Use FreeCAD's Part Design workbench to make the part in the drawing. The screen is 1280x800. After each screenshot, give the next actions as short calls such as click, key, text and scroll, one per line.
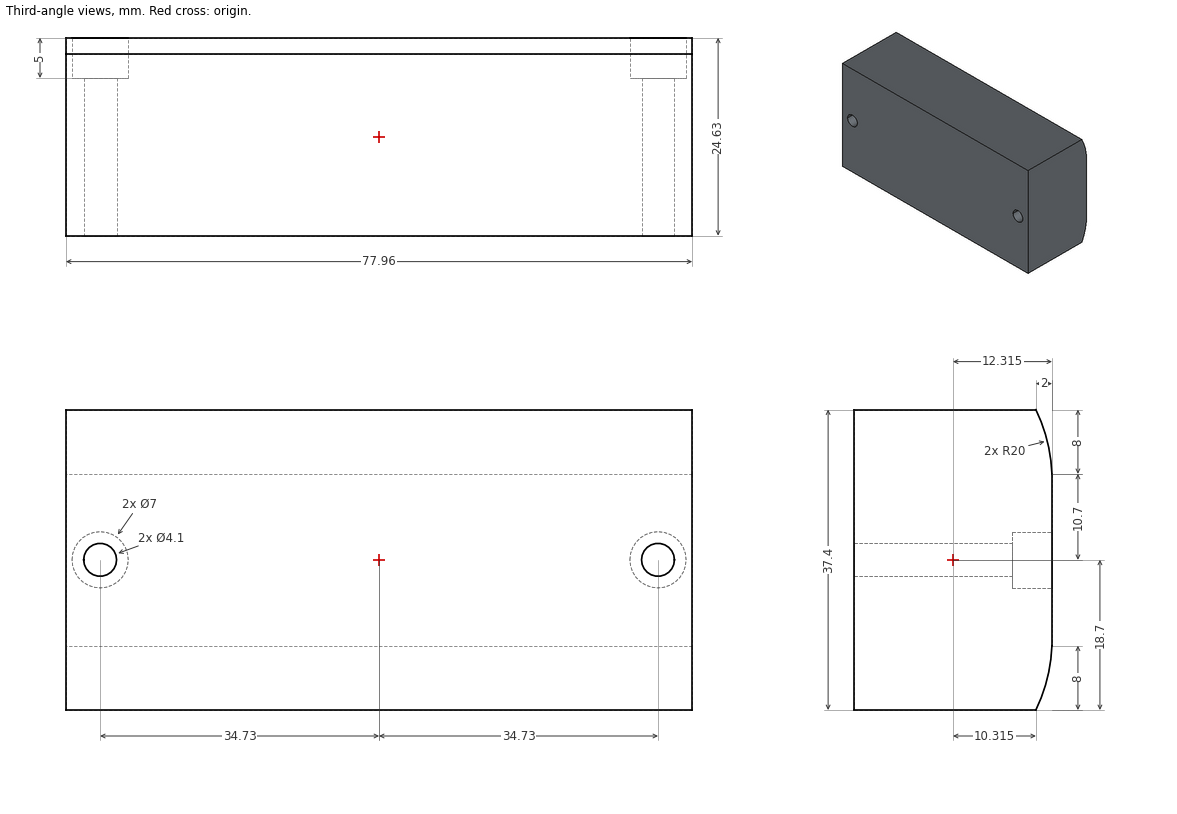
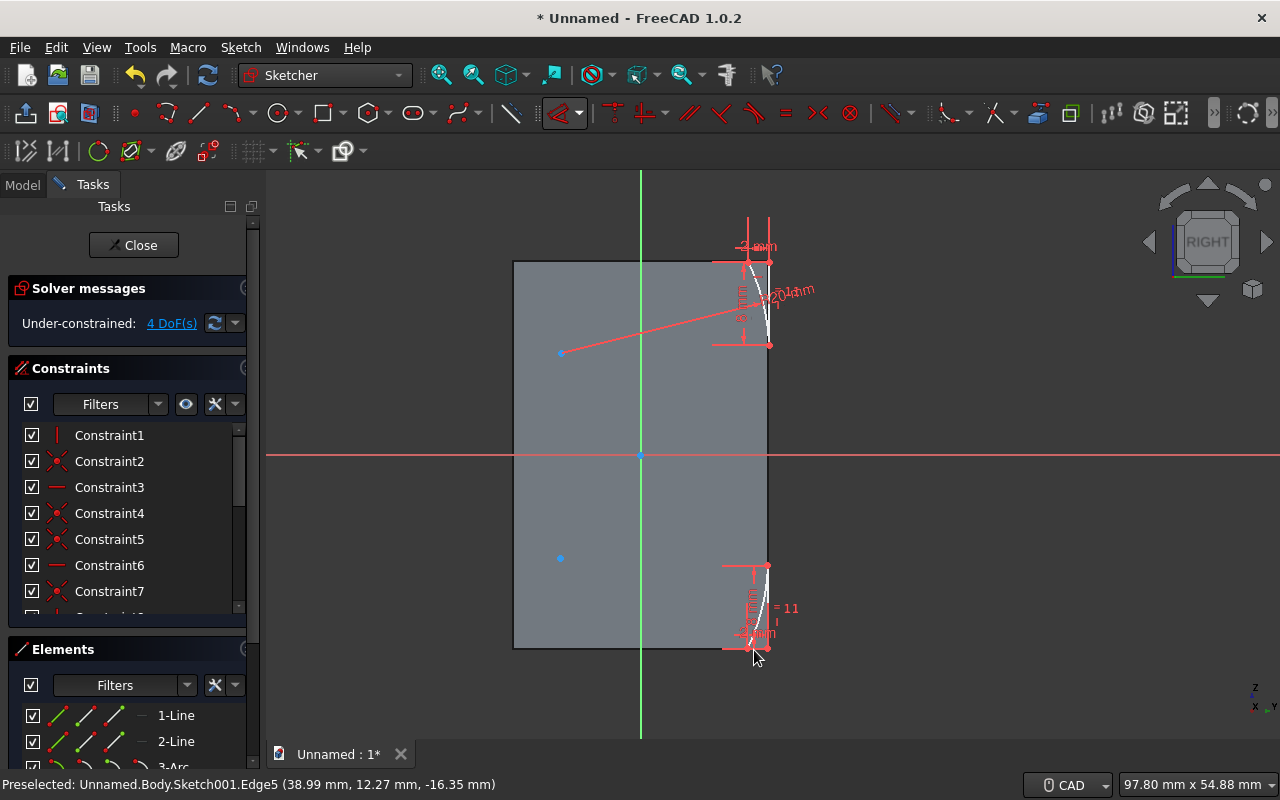
click(769, 345)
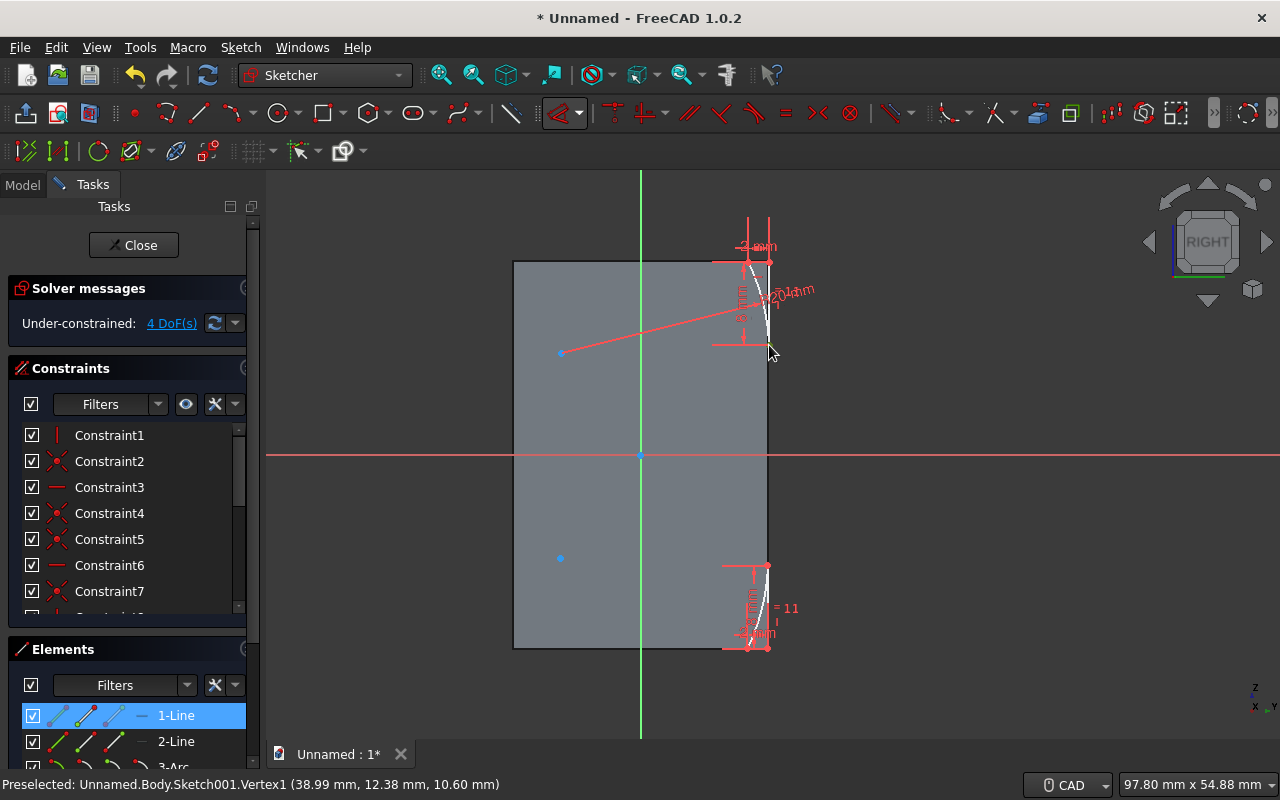
click(582, 114)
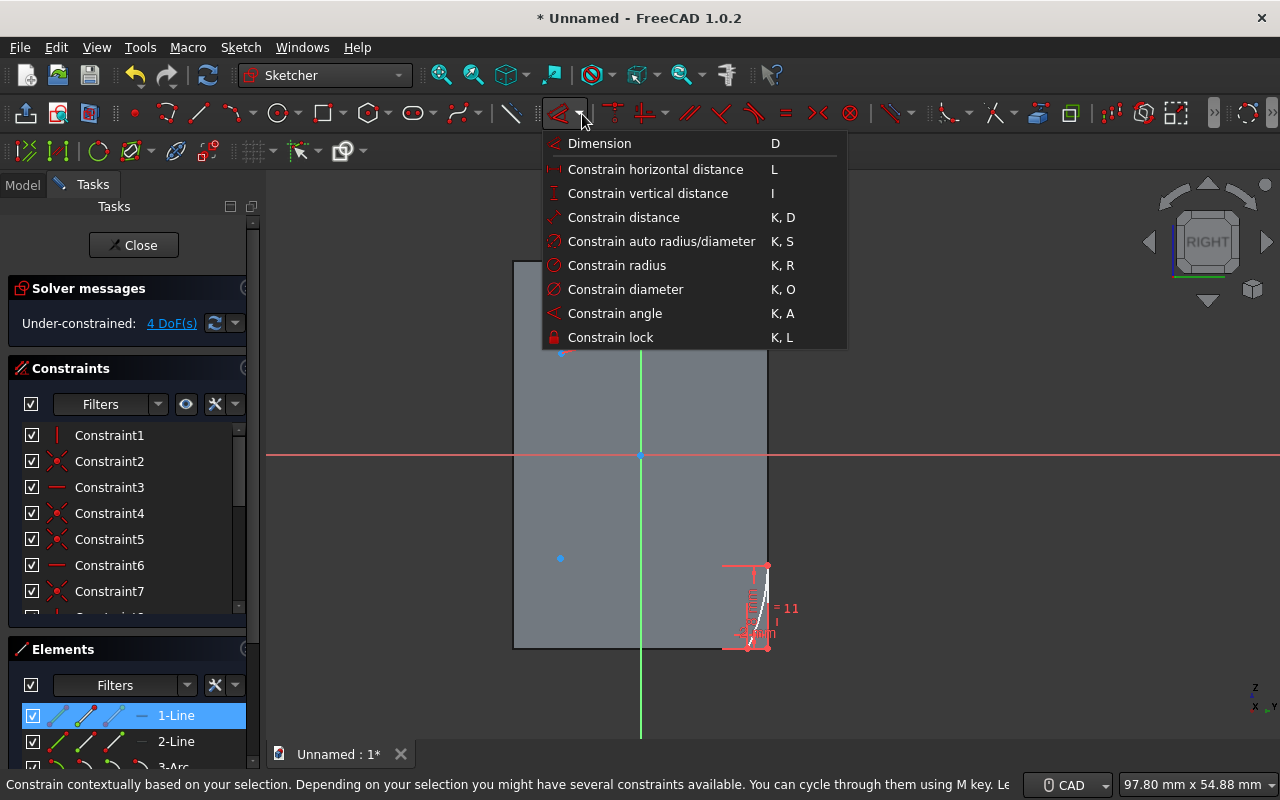
click(695, 193)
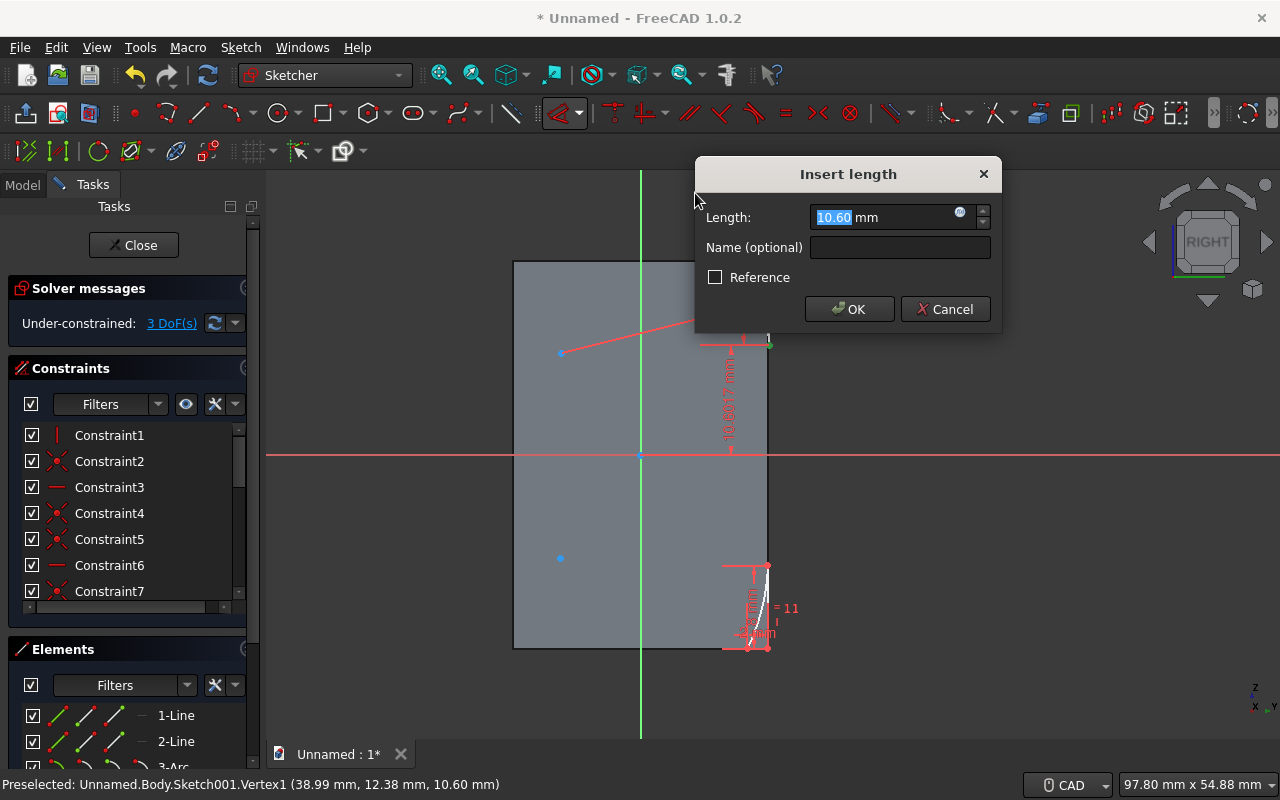
text(10.7)
key(Return)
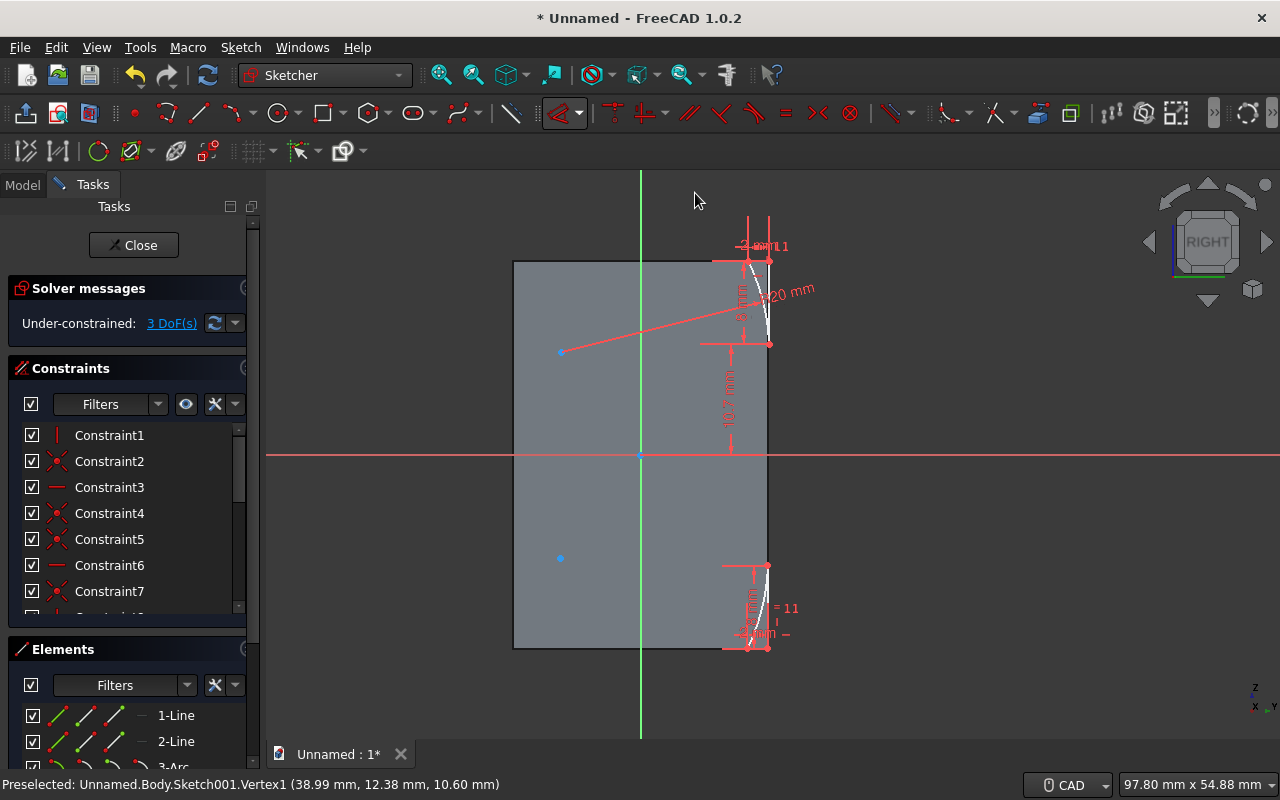
click(747, 649)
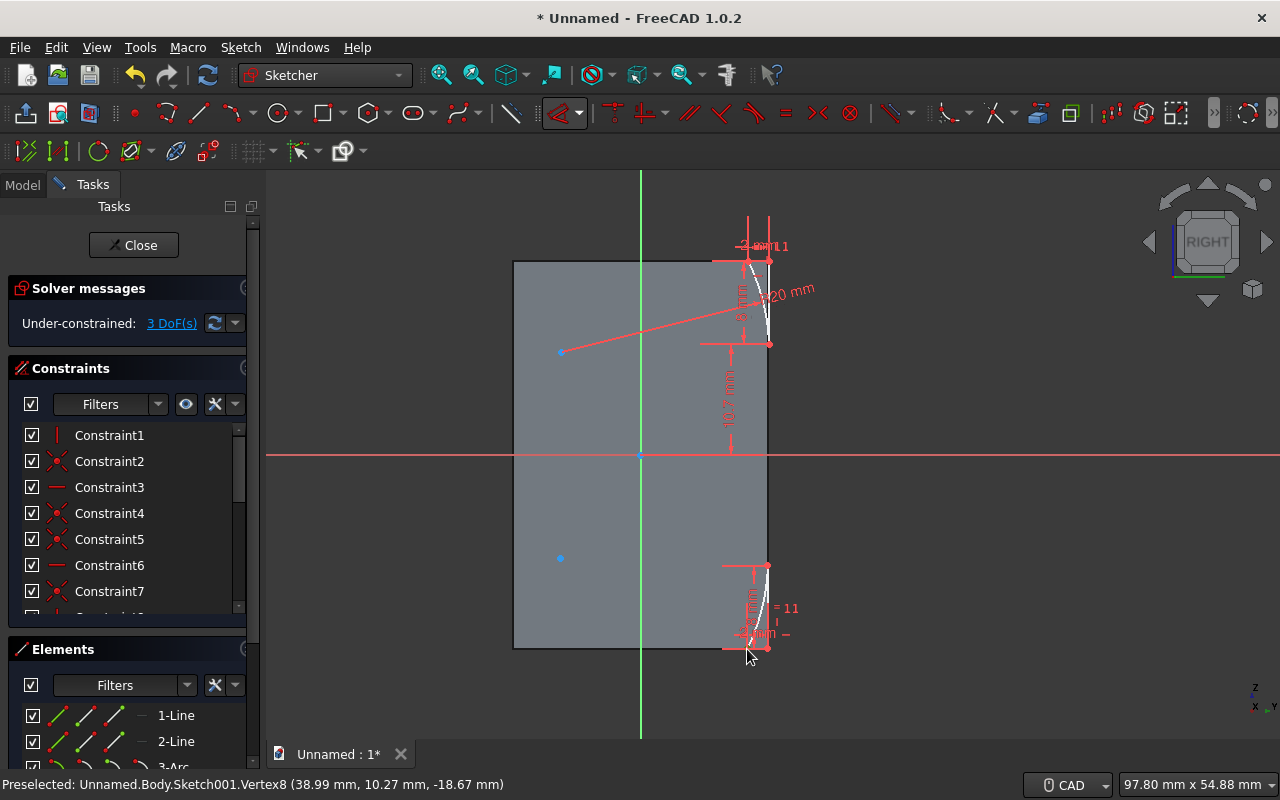
click(582, 114)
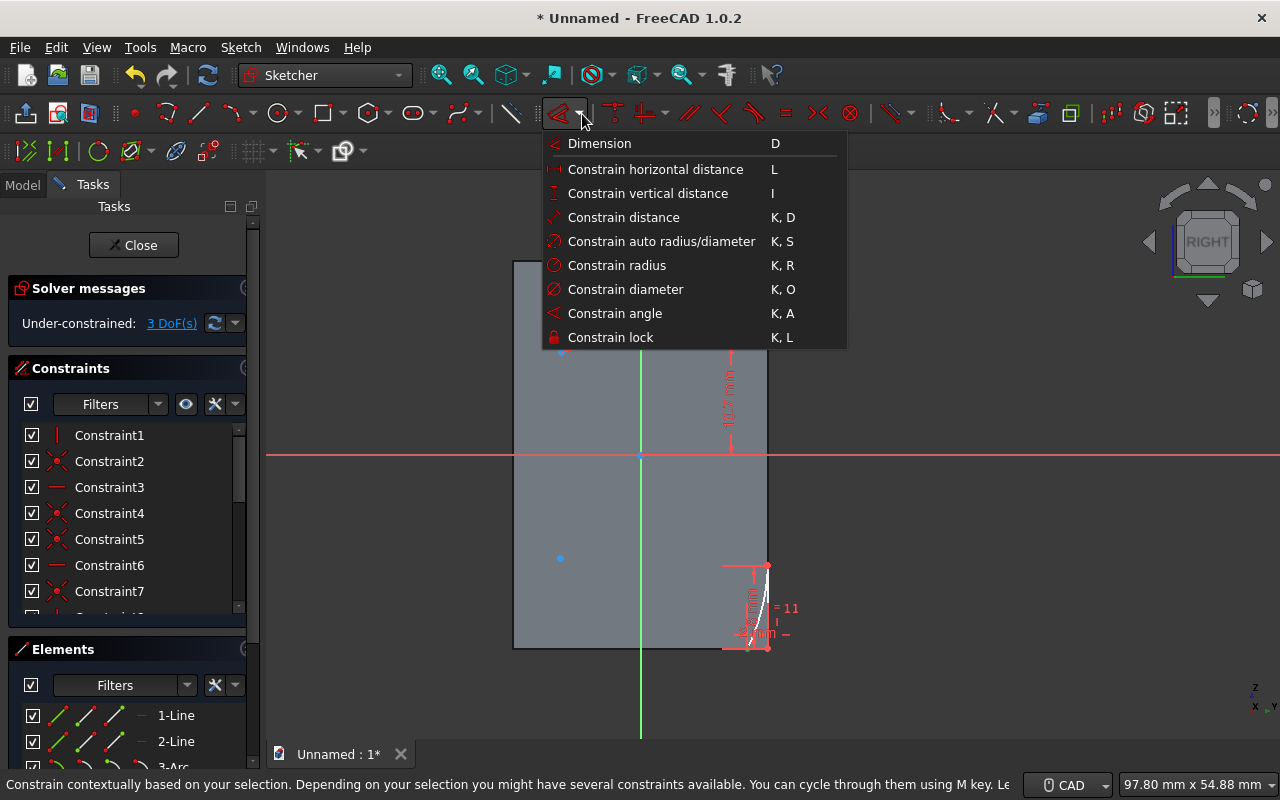
click(695, 193)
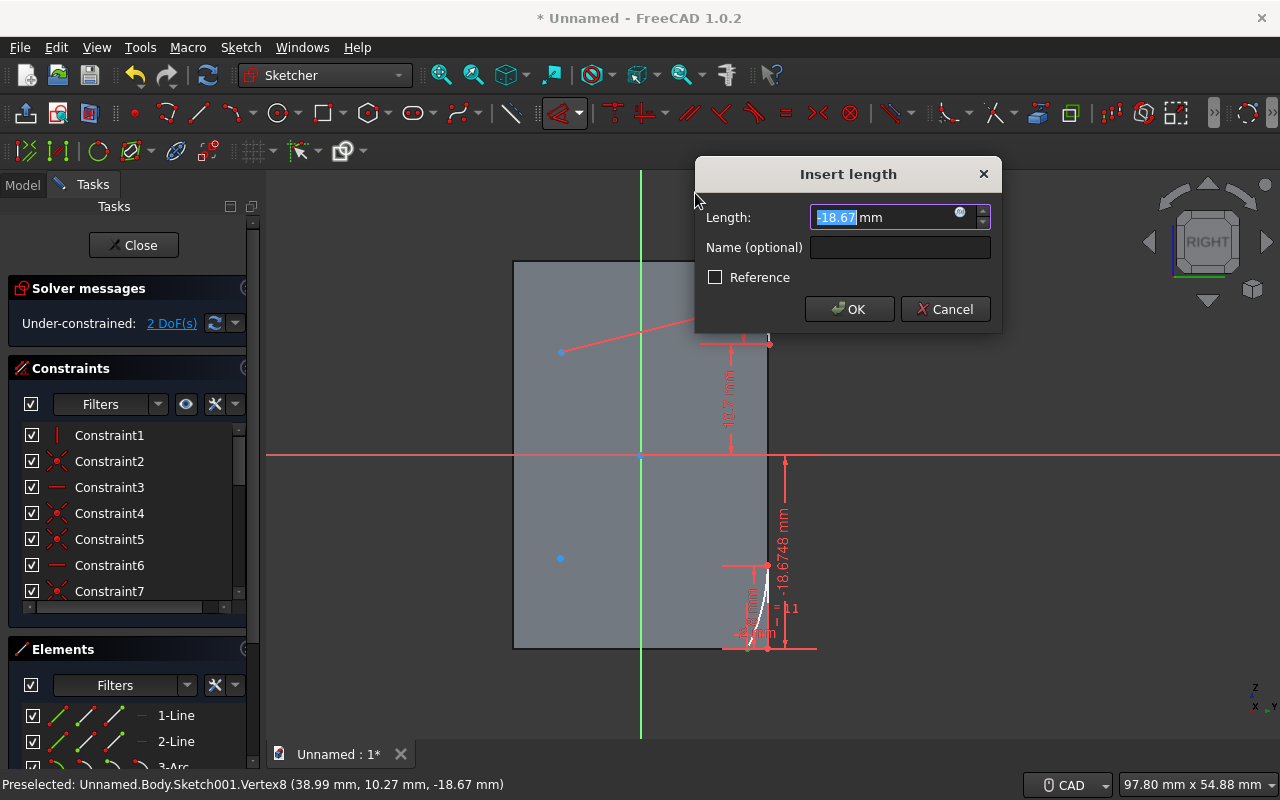
text(-18.7)
key(Return)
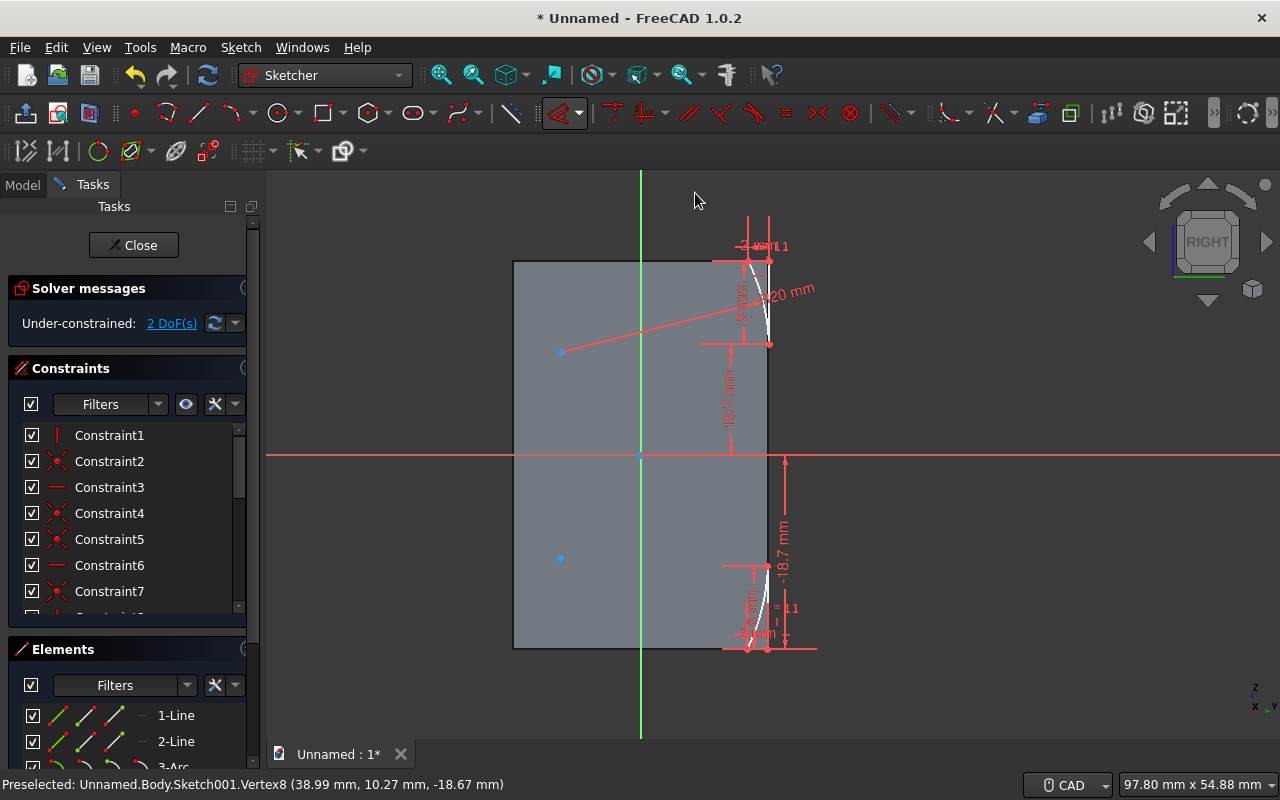
click(769, 344)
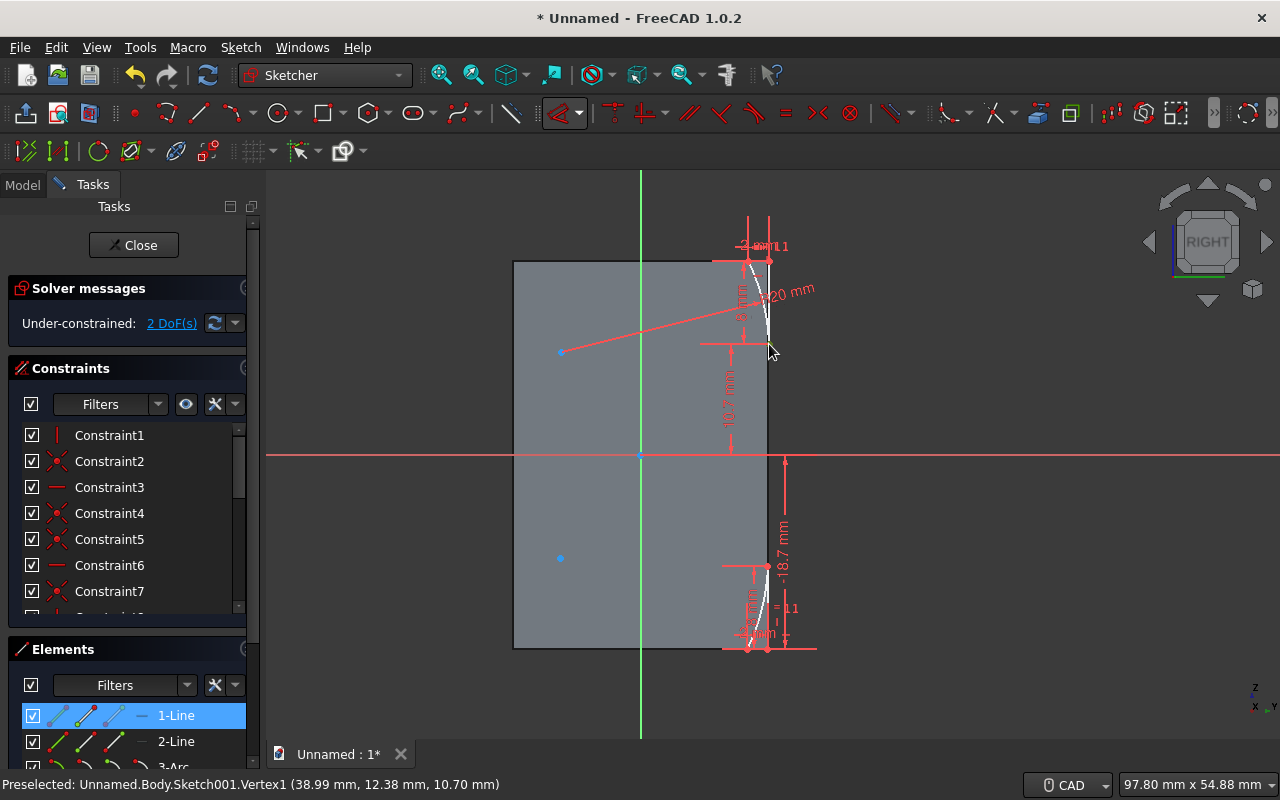
click(582, 114)